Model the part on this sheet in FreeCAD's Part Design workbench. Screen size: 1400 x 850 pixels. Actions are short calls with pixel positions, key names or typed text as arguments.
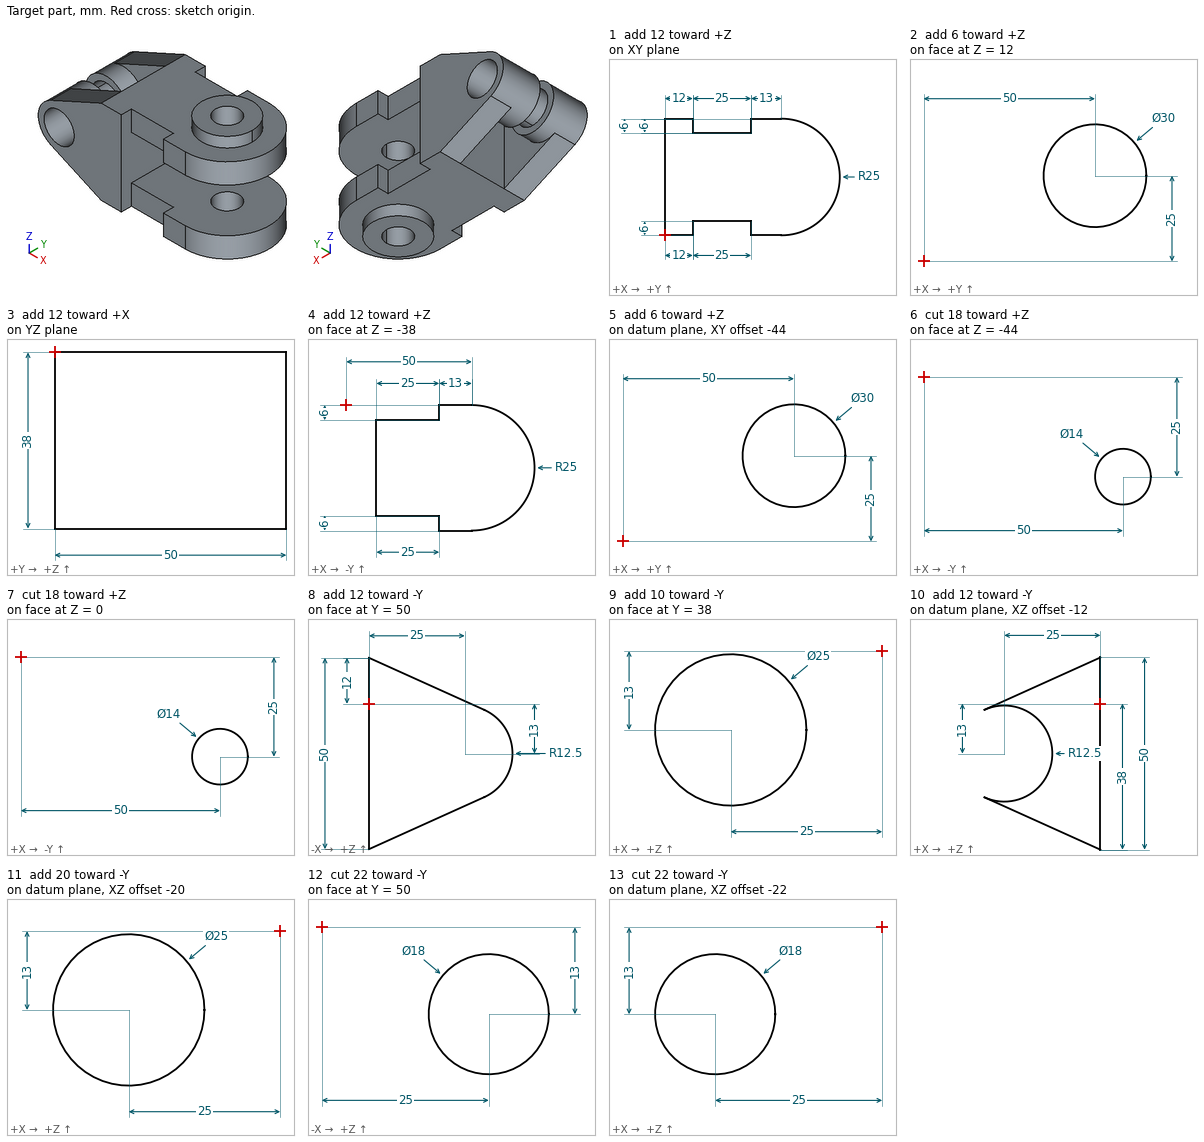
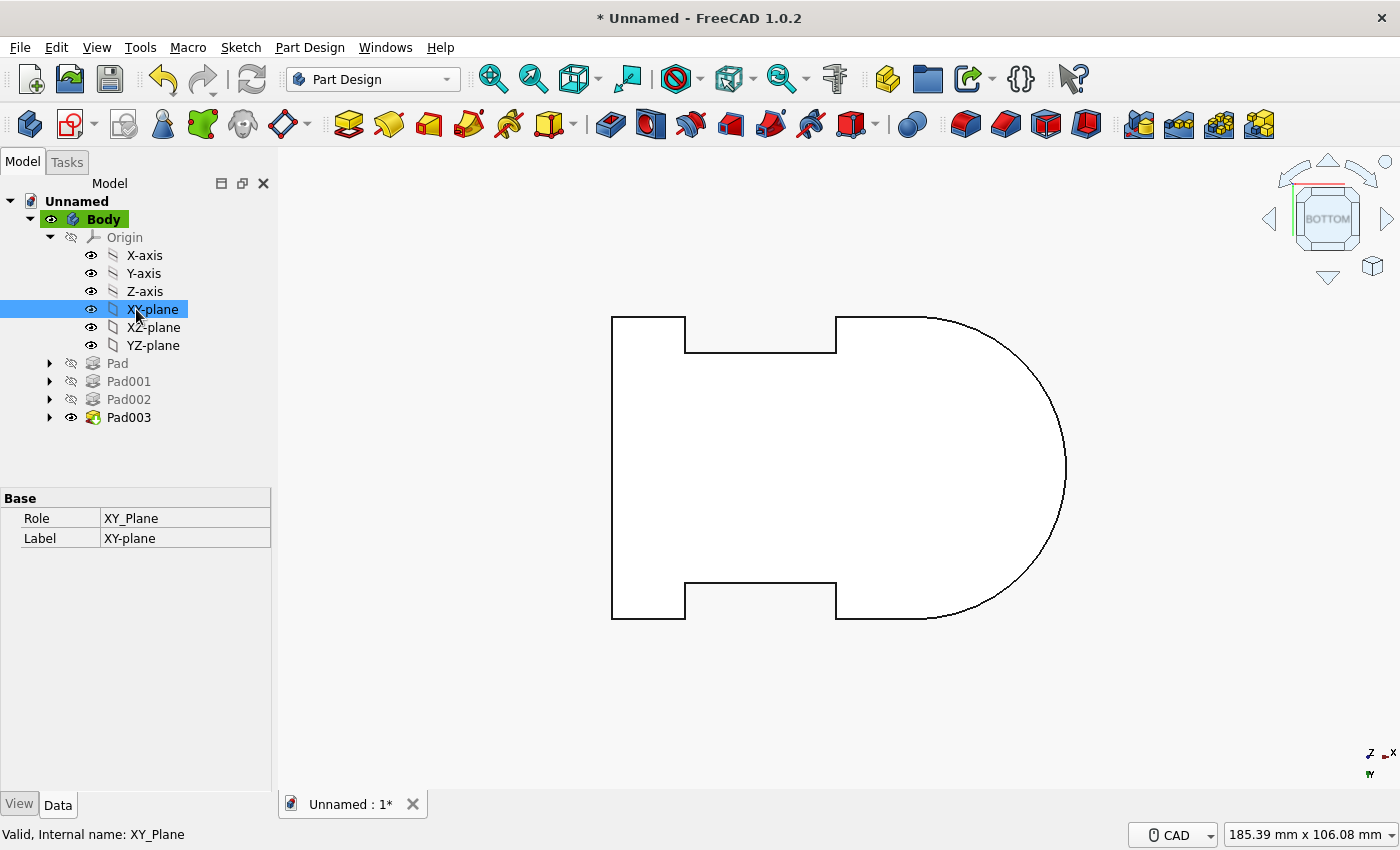
click(284, 124)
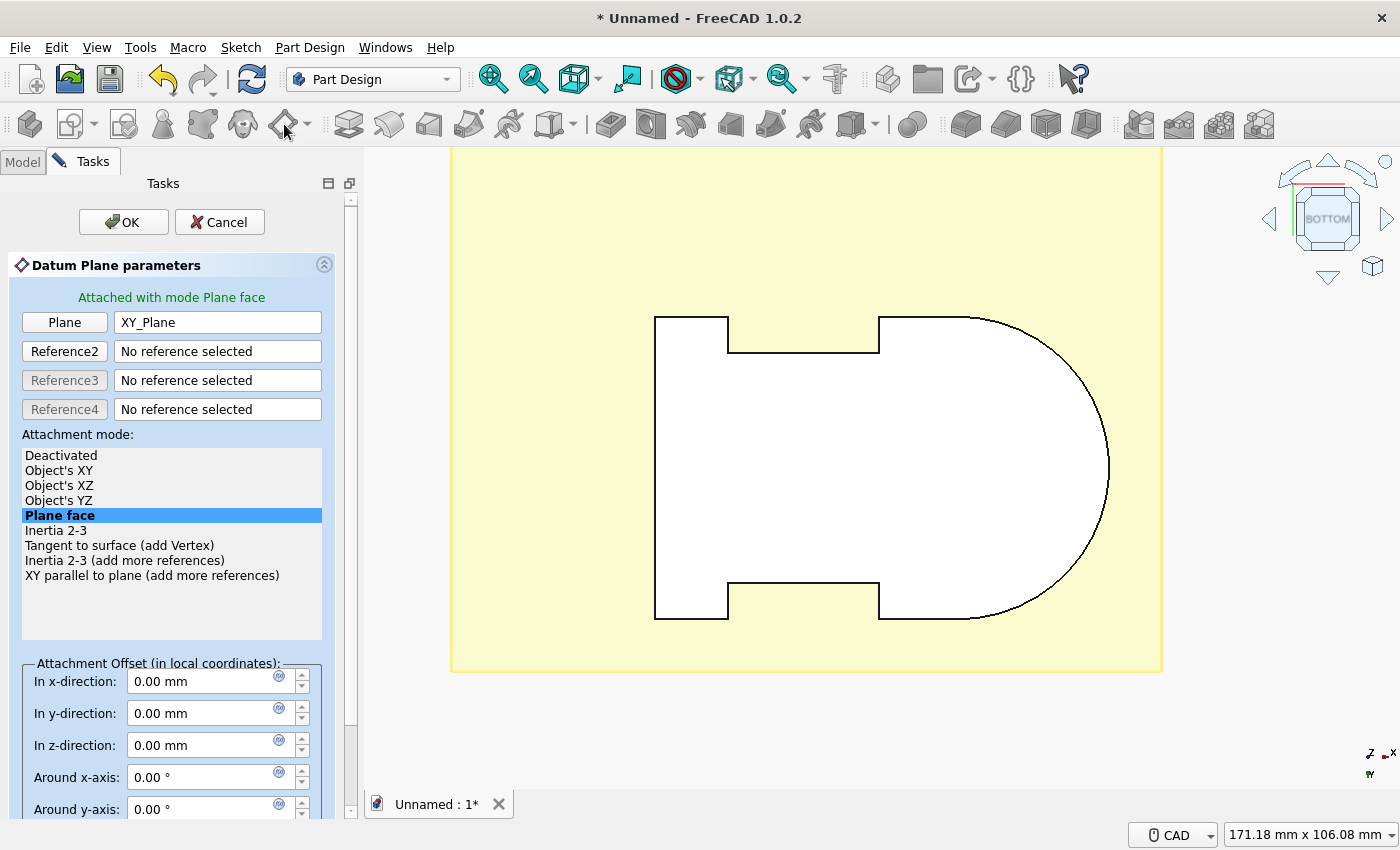
triple_click(210, 745)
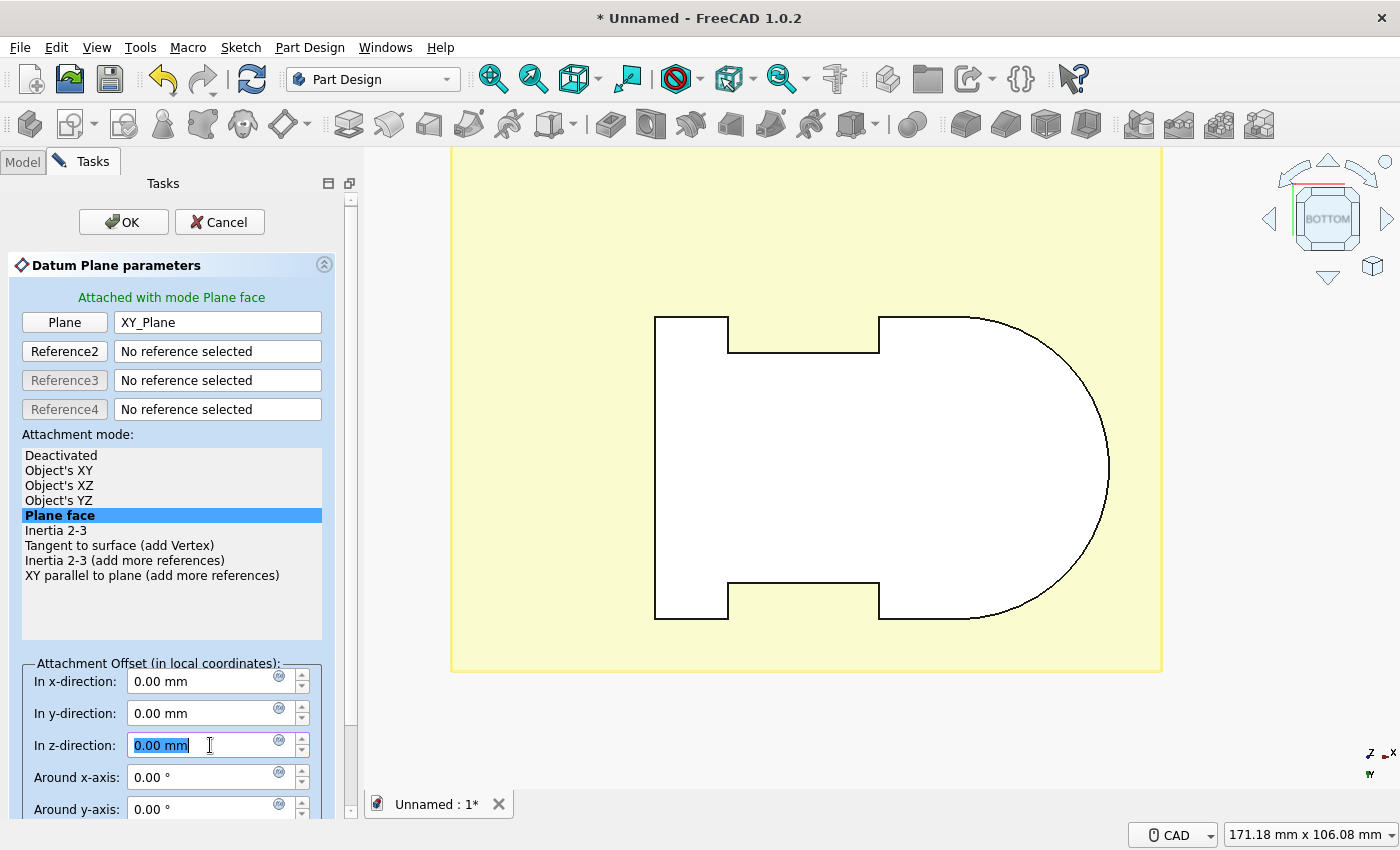
text(-44)
key(Tab)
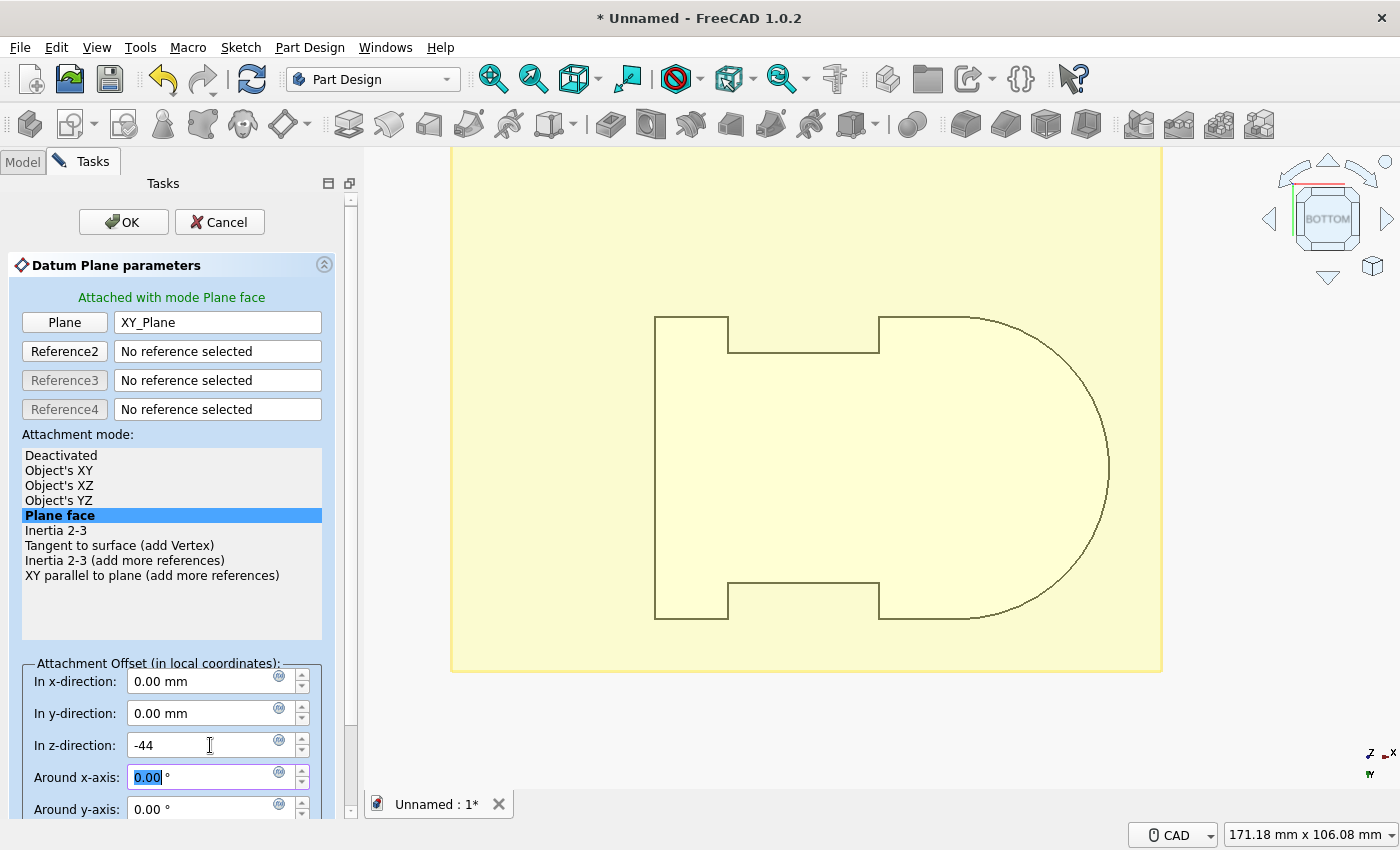
click(124, 222)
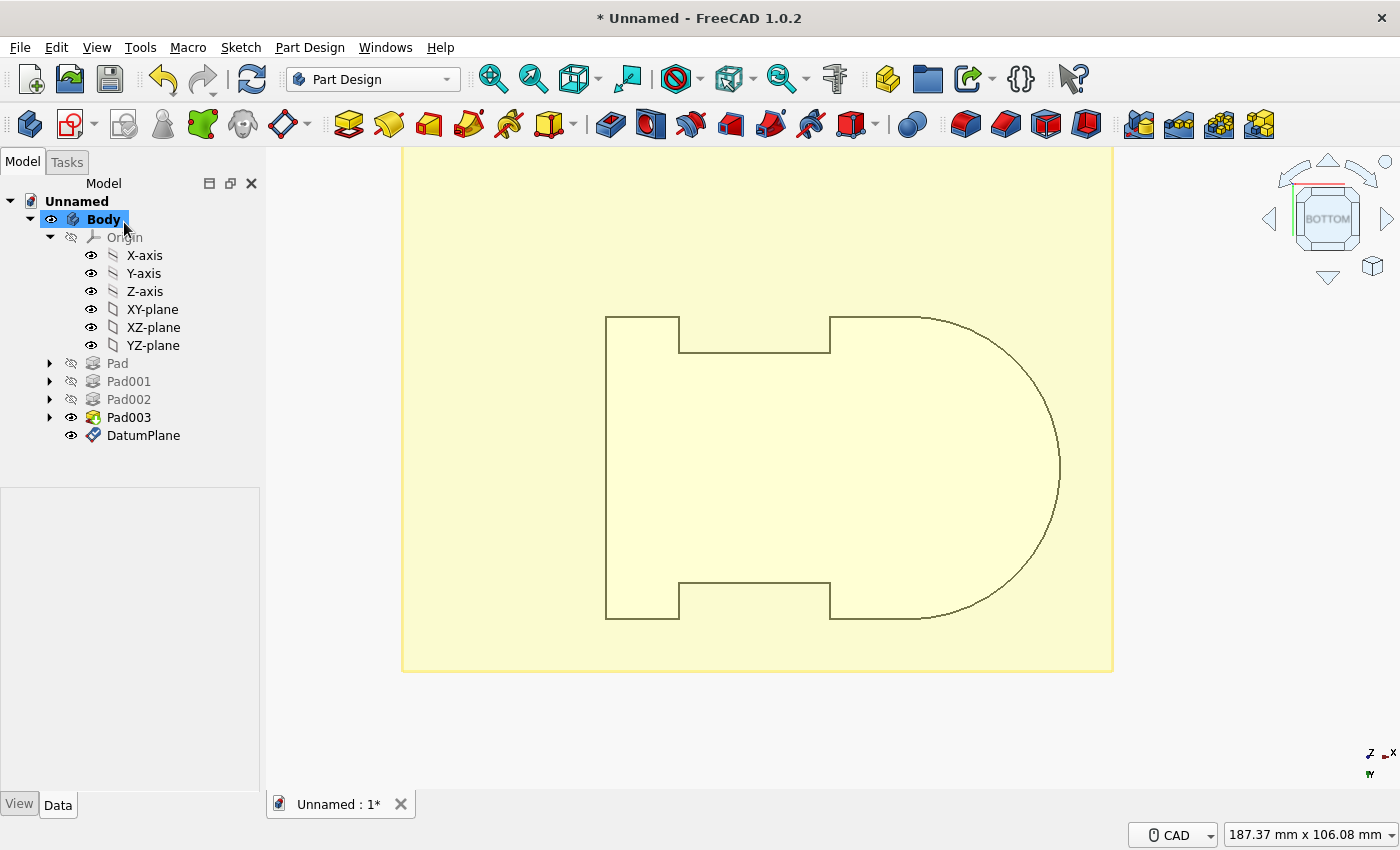
click(116, 435)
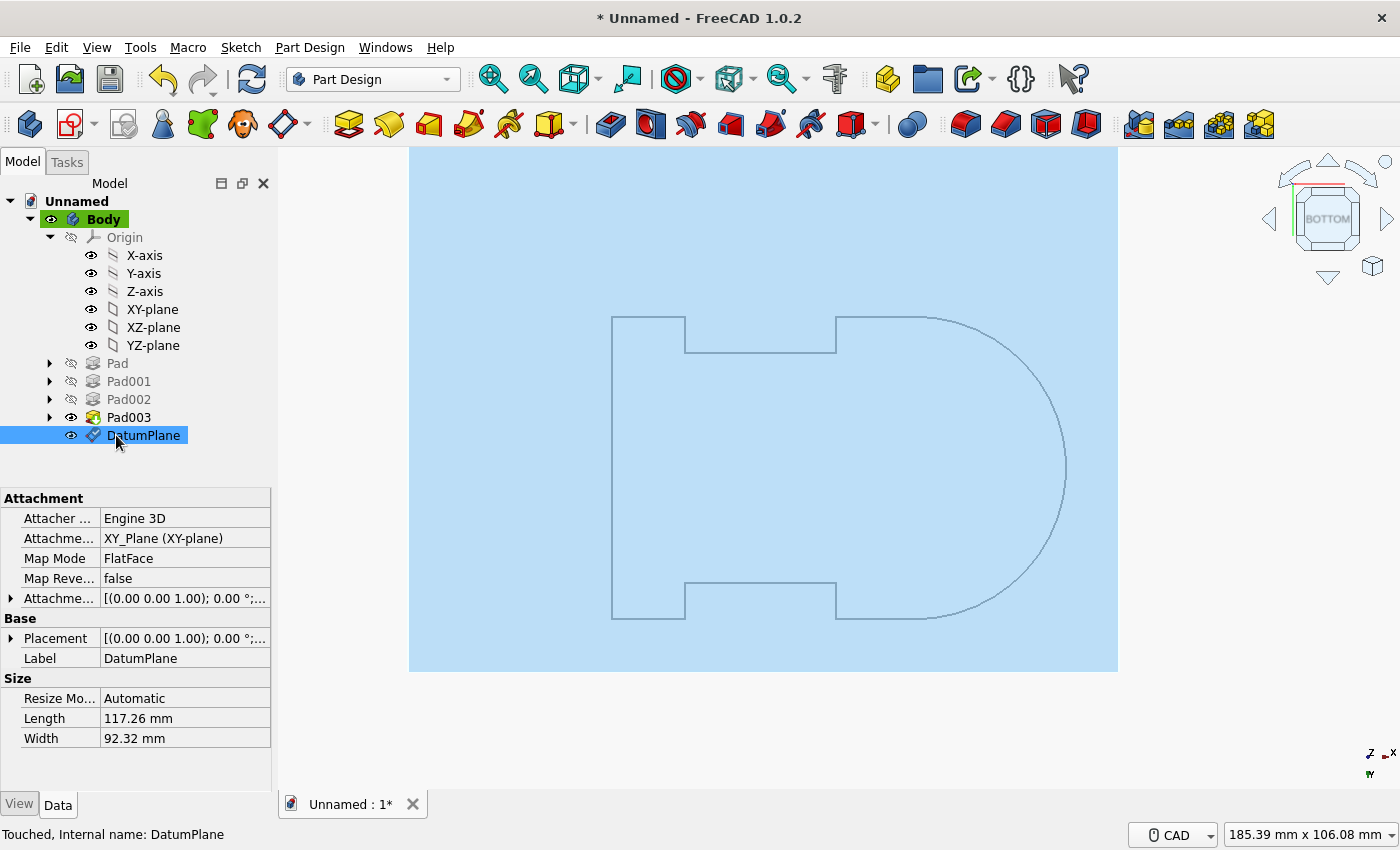
click(70, 124)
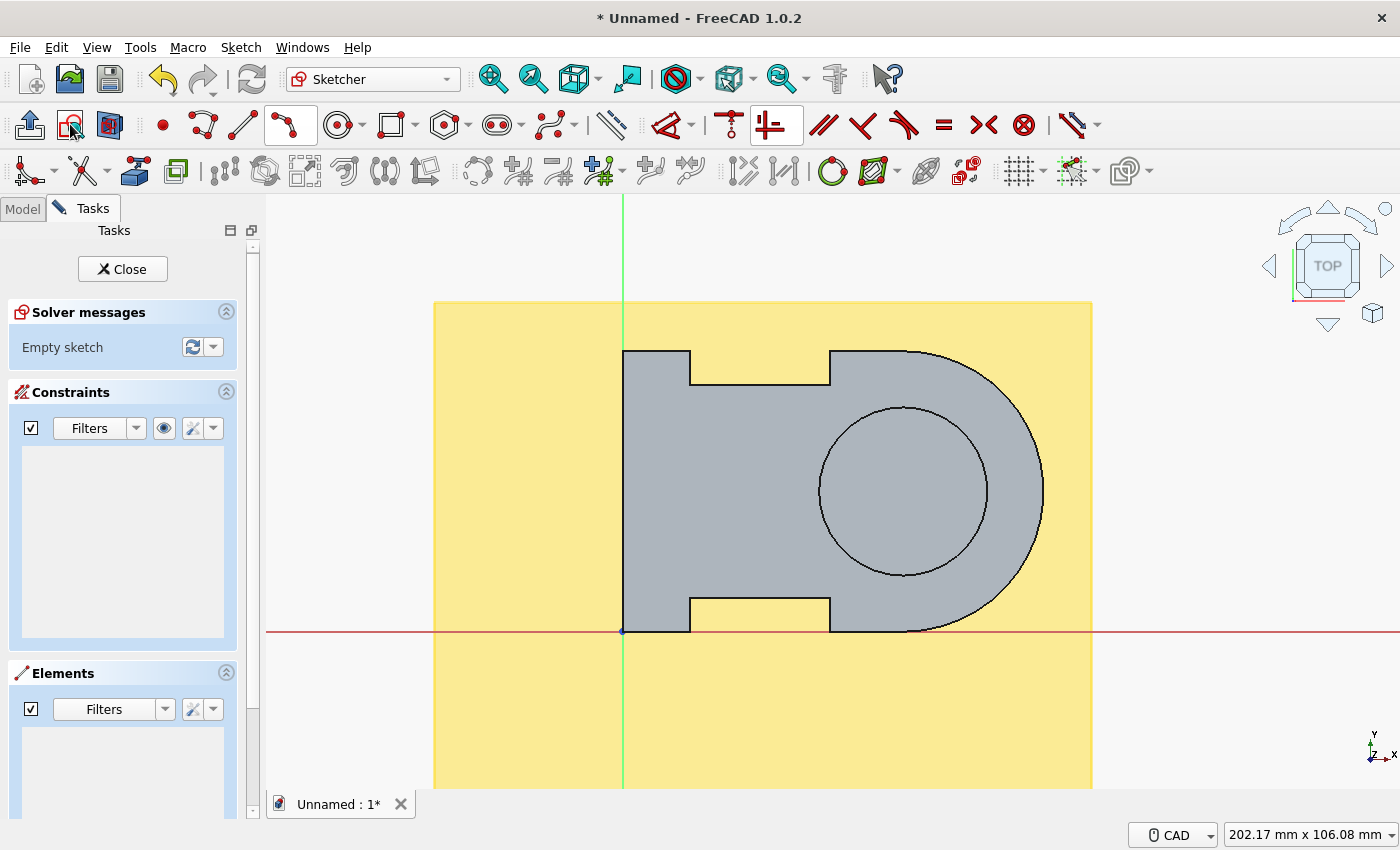
key(q)
key(s)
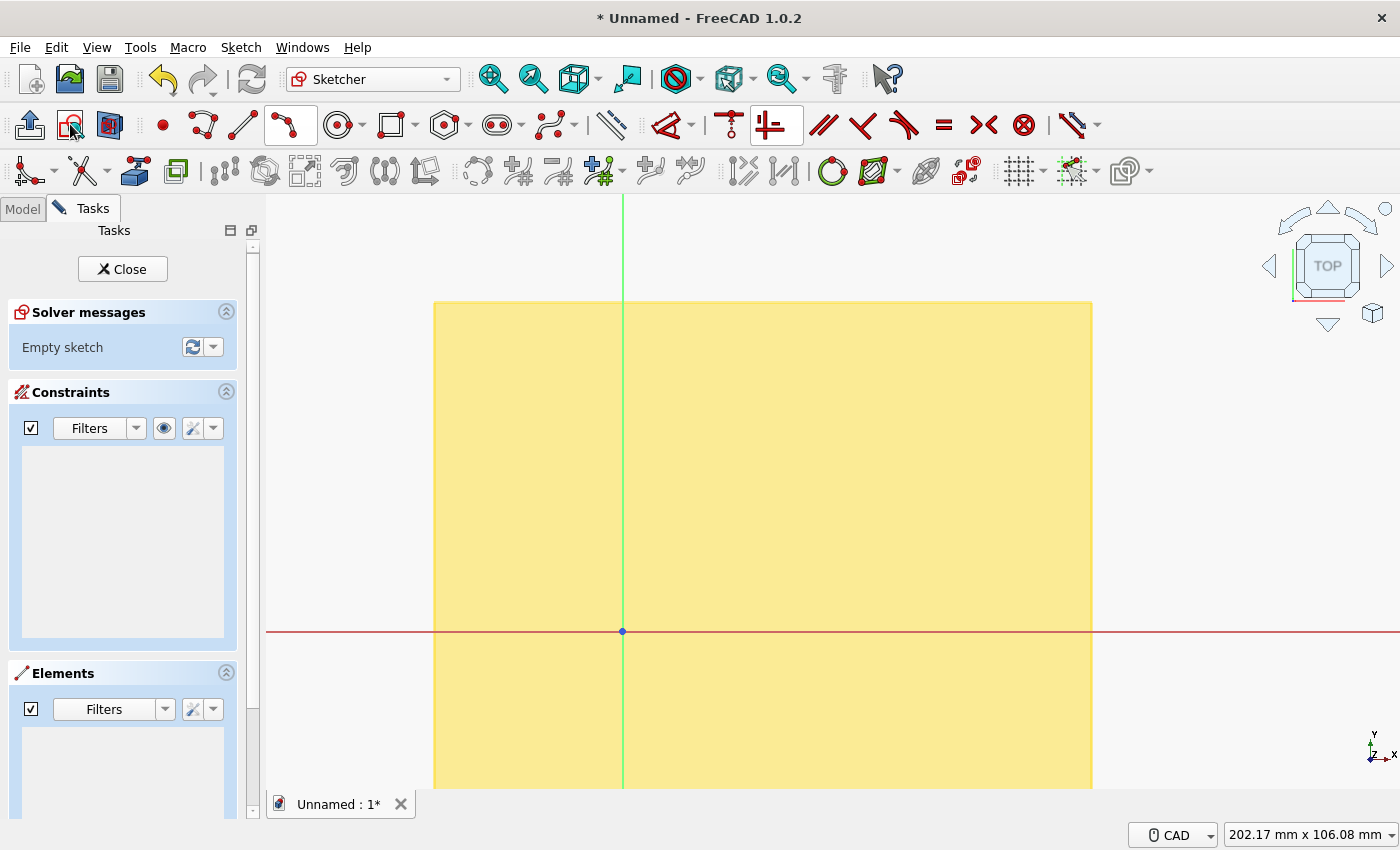
scroll(855, 554, up, 3)